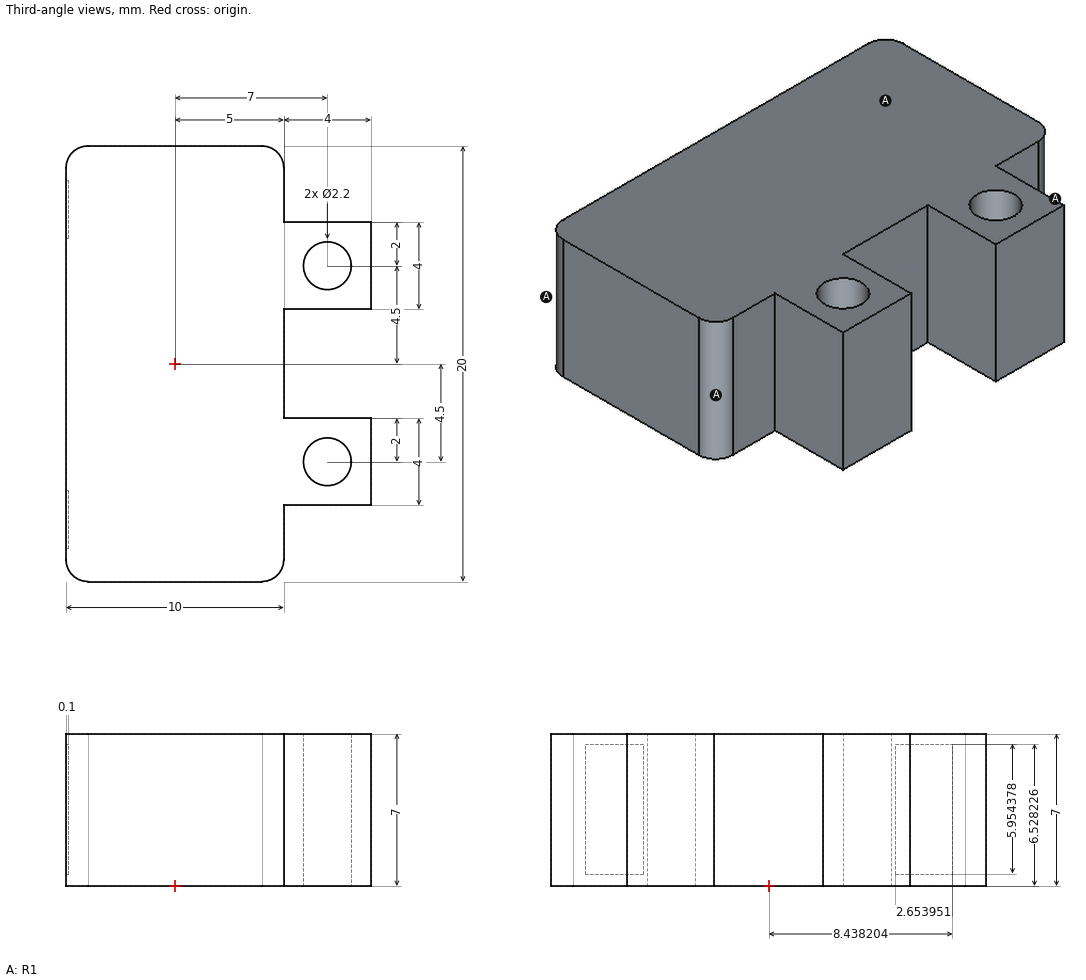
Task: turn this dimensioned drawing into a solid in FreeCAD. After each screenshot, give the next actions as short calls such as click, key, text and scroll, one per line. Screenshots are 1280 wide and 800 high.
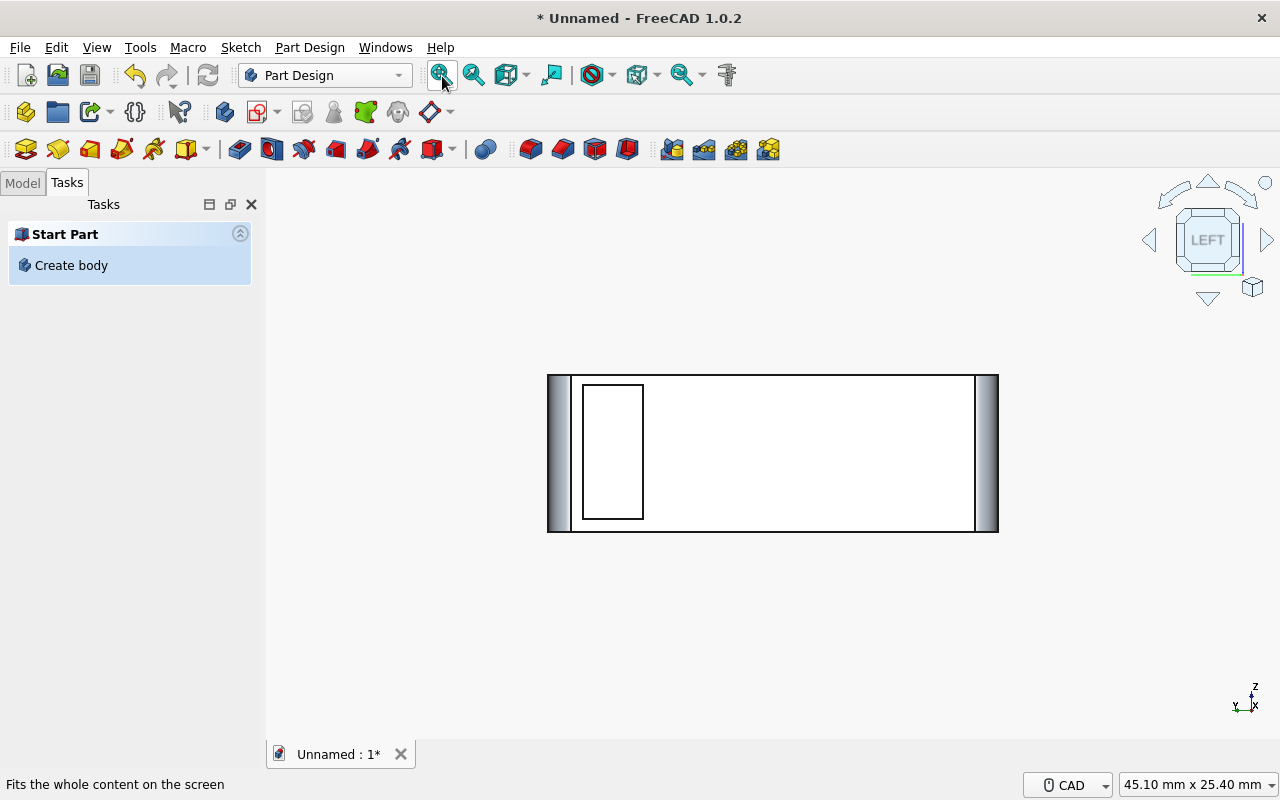
click(23, 182)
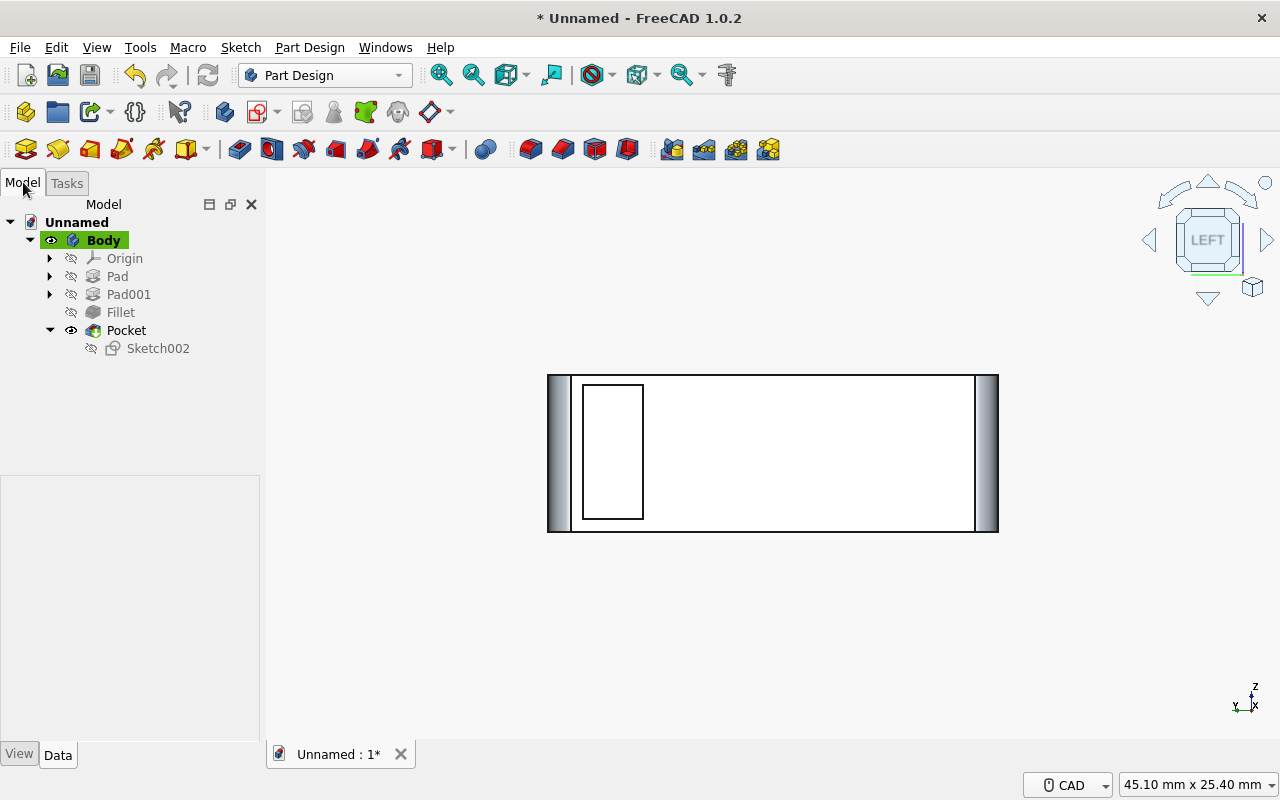
click(116, 330)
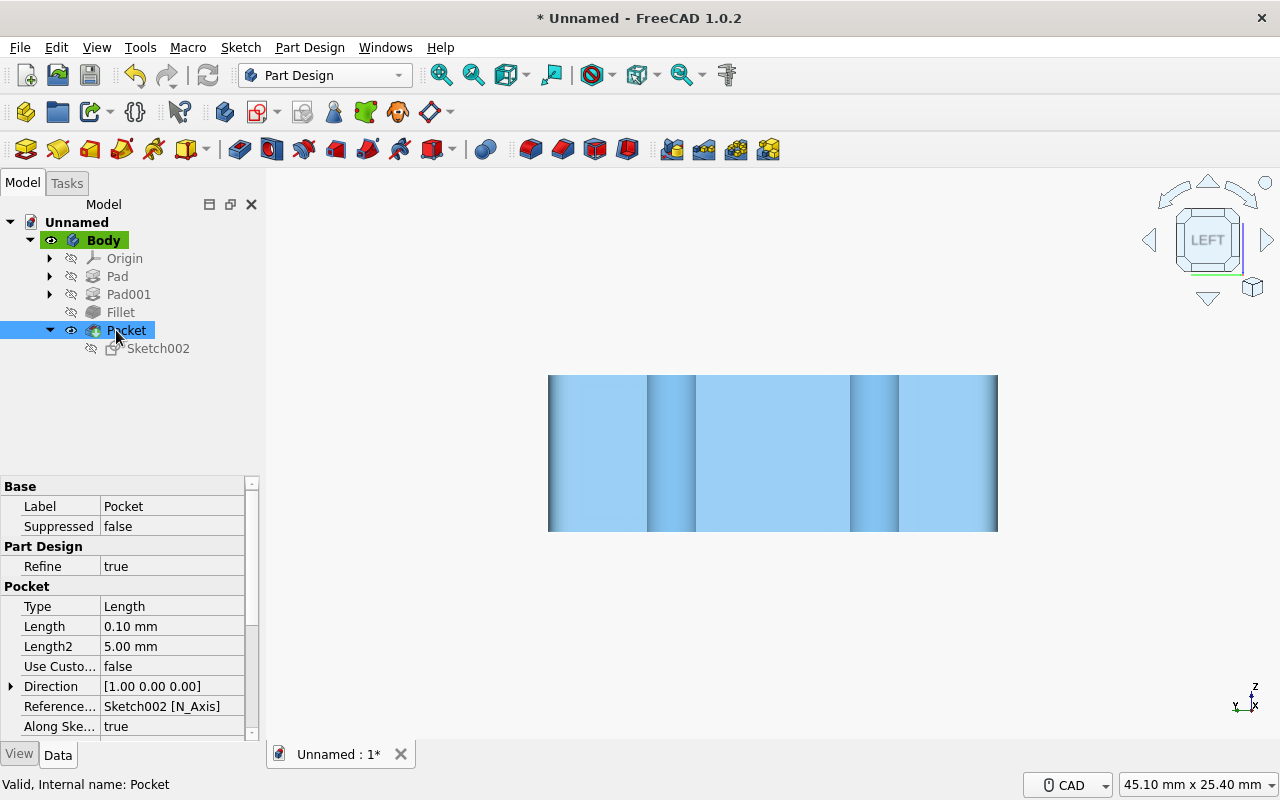
click(672, 150)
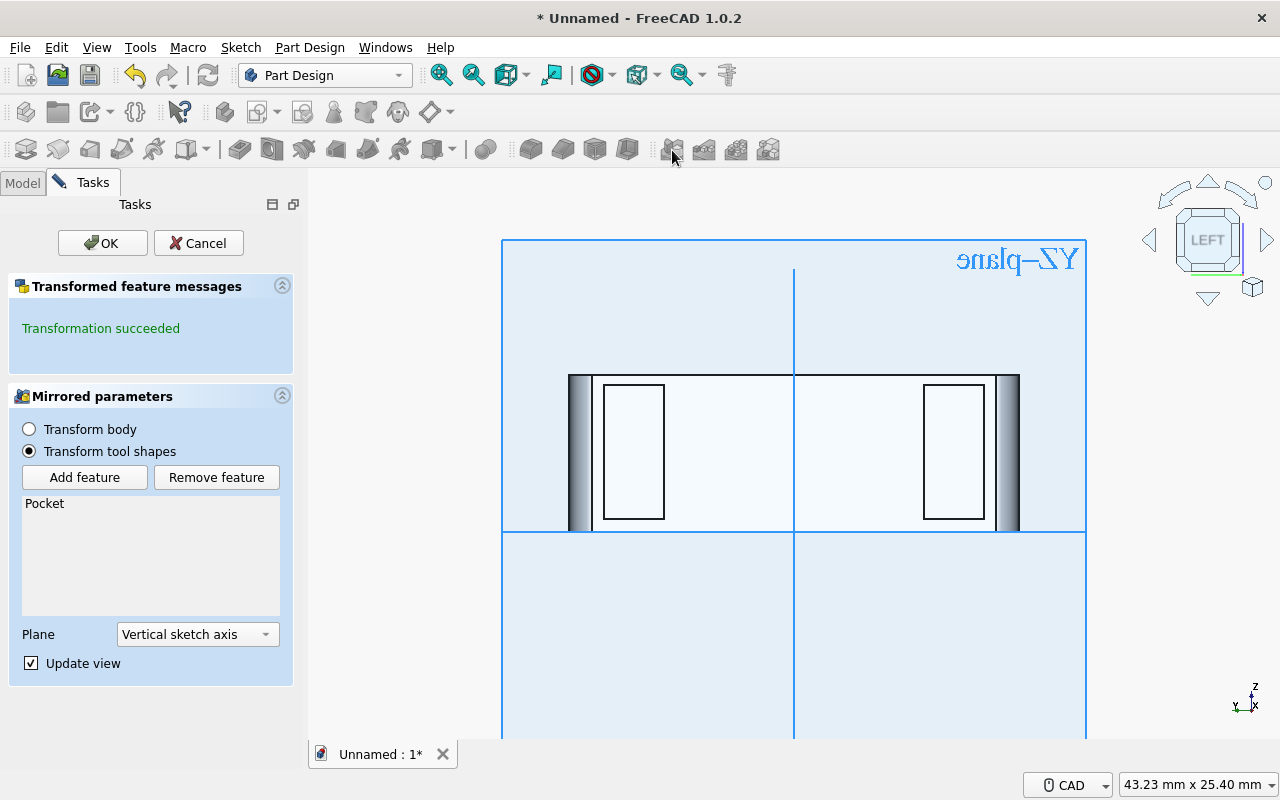
click(198, 634)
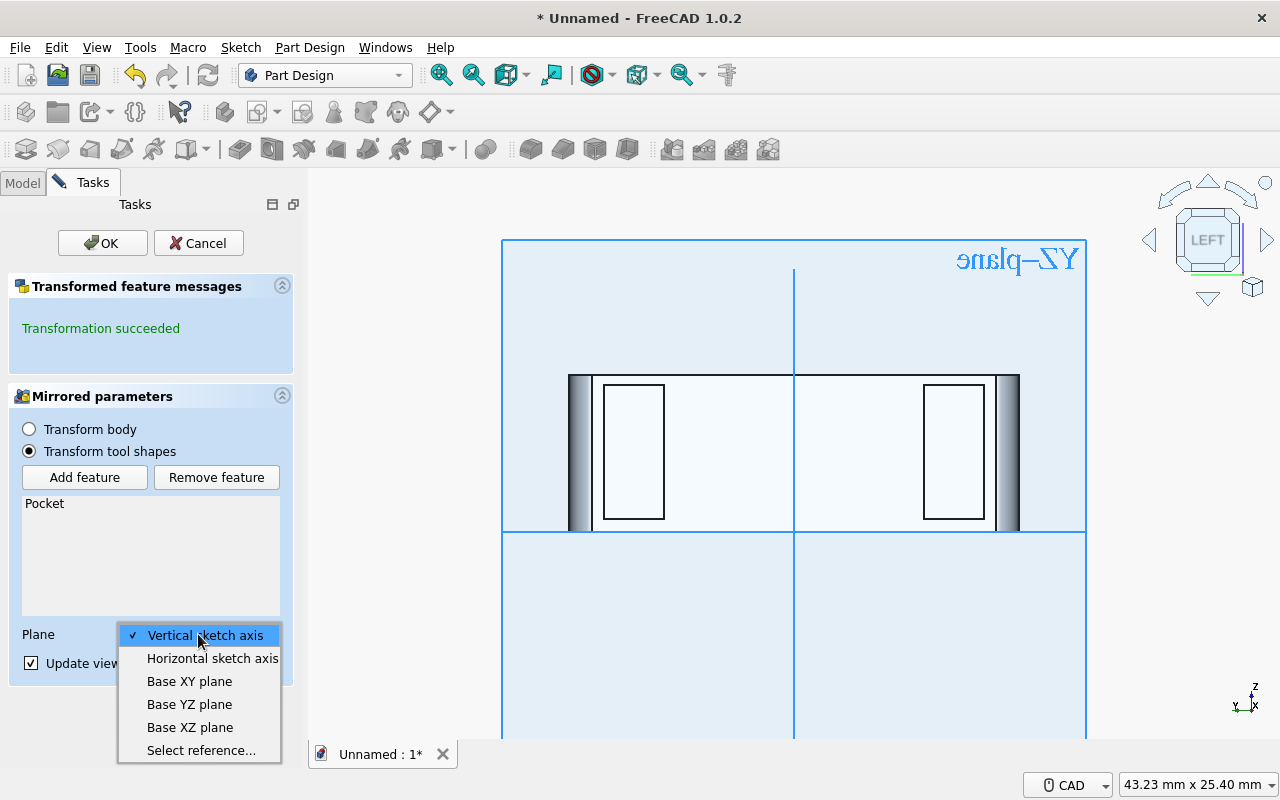
click(198, 728)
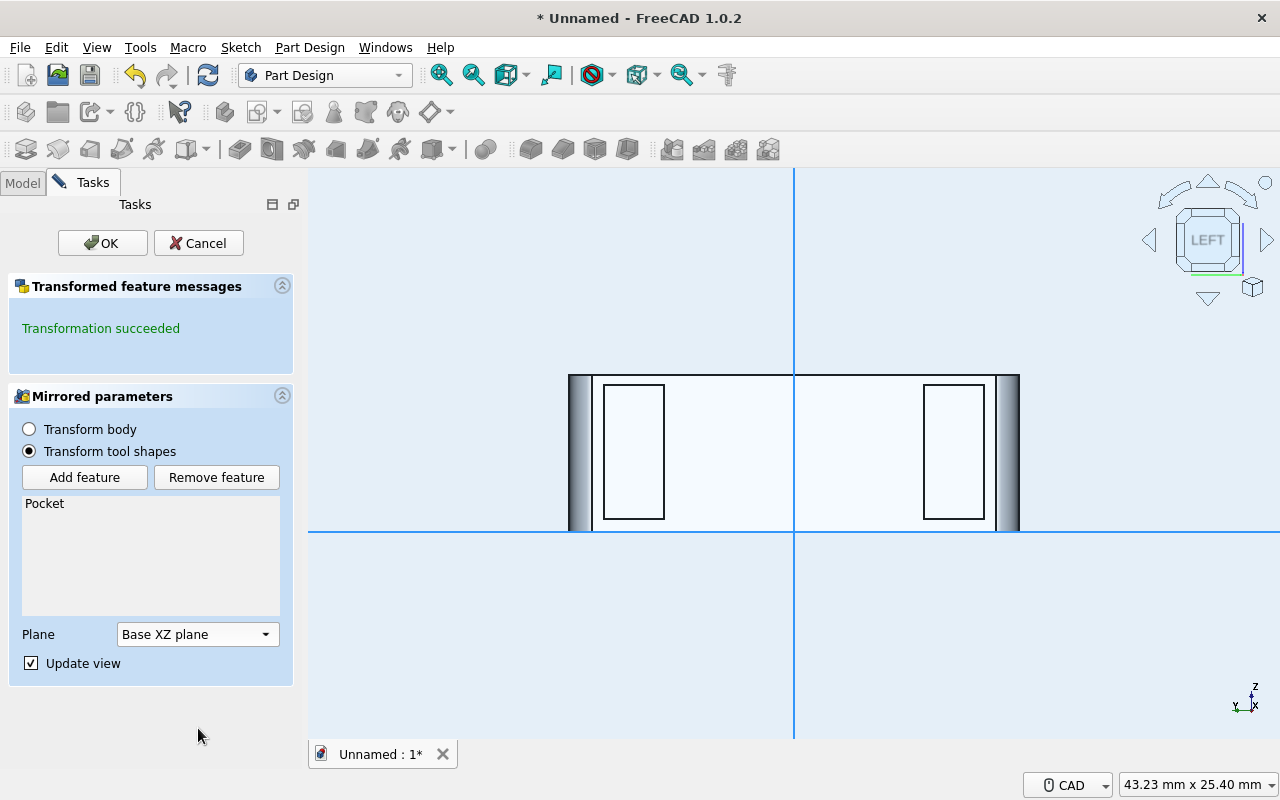
click(103, 243)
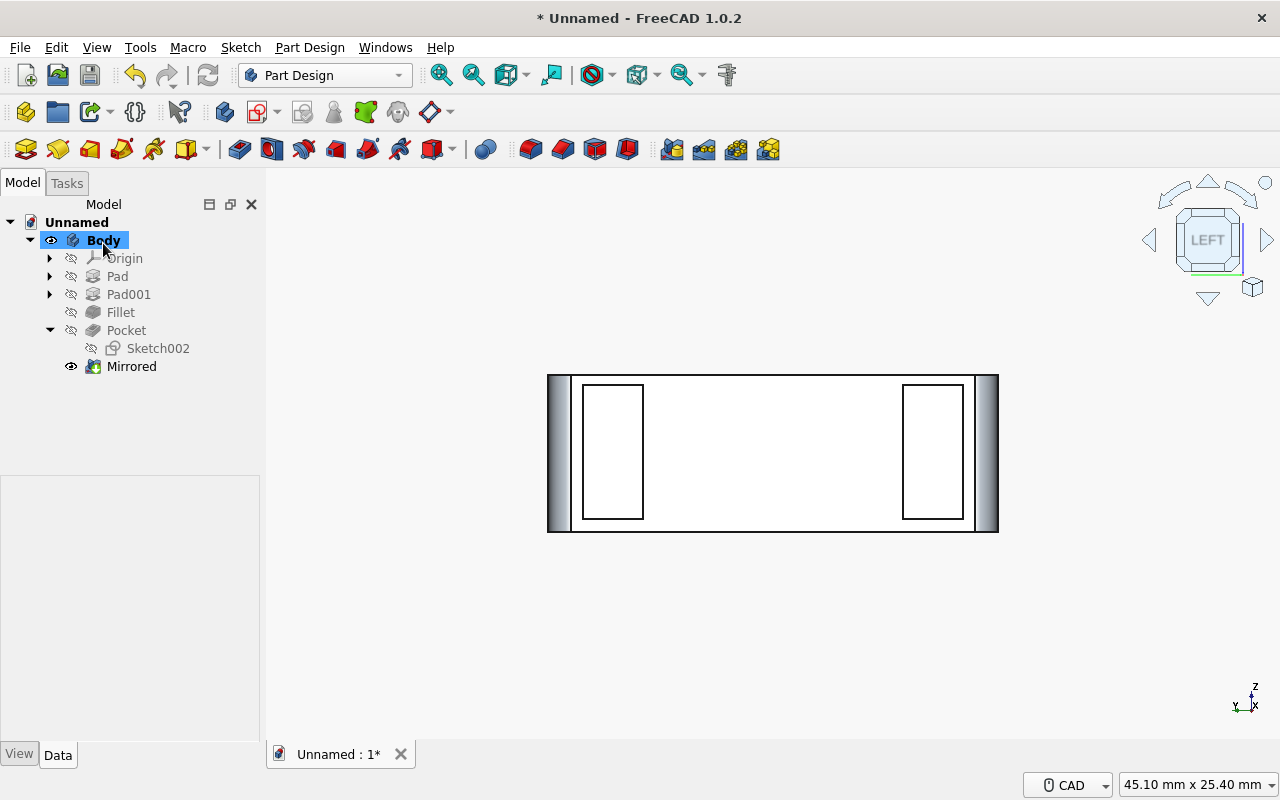
key(0)